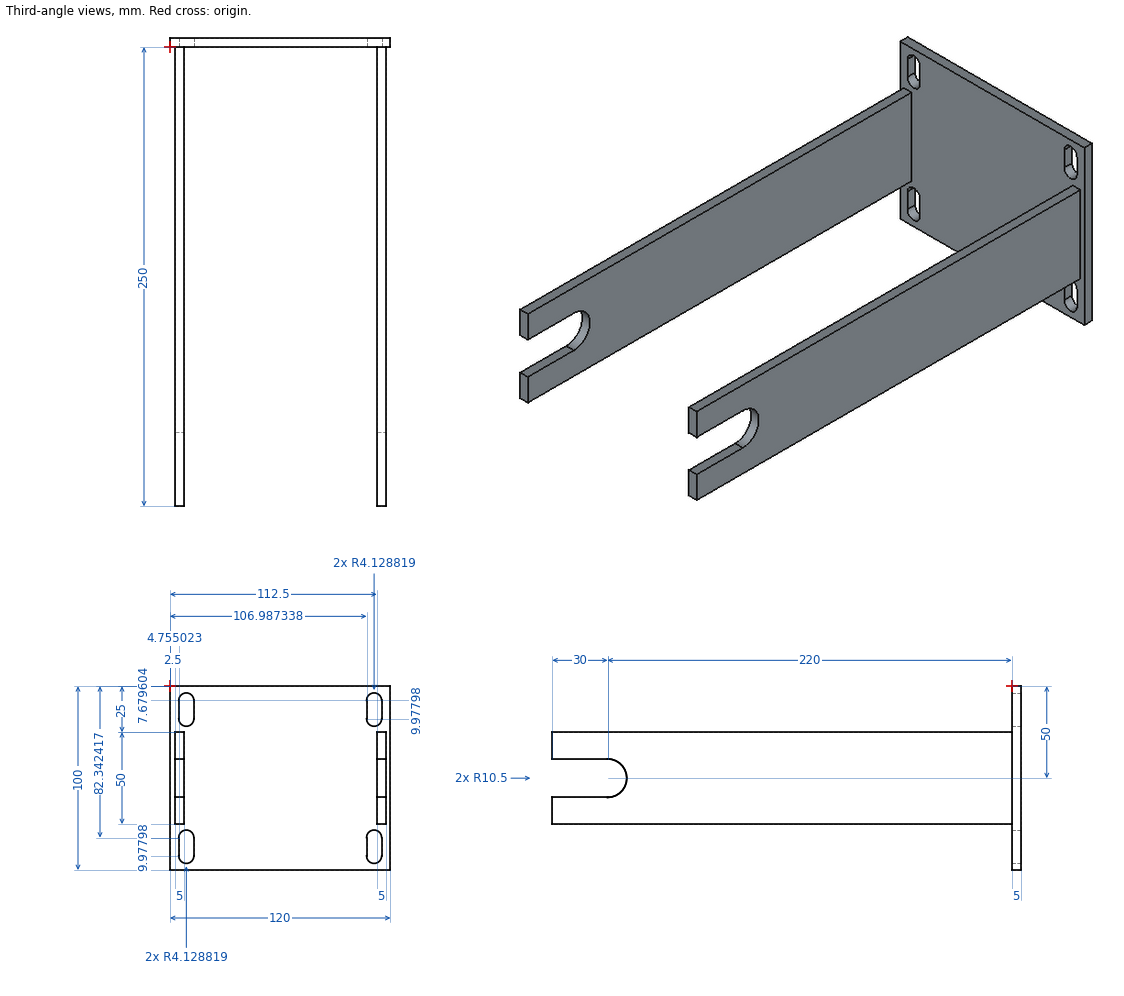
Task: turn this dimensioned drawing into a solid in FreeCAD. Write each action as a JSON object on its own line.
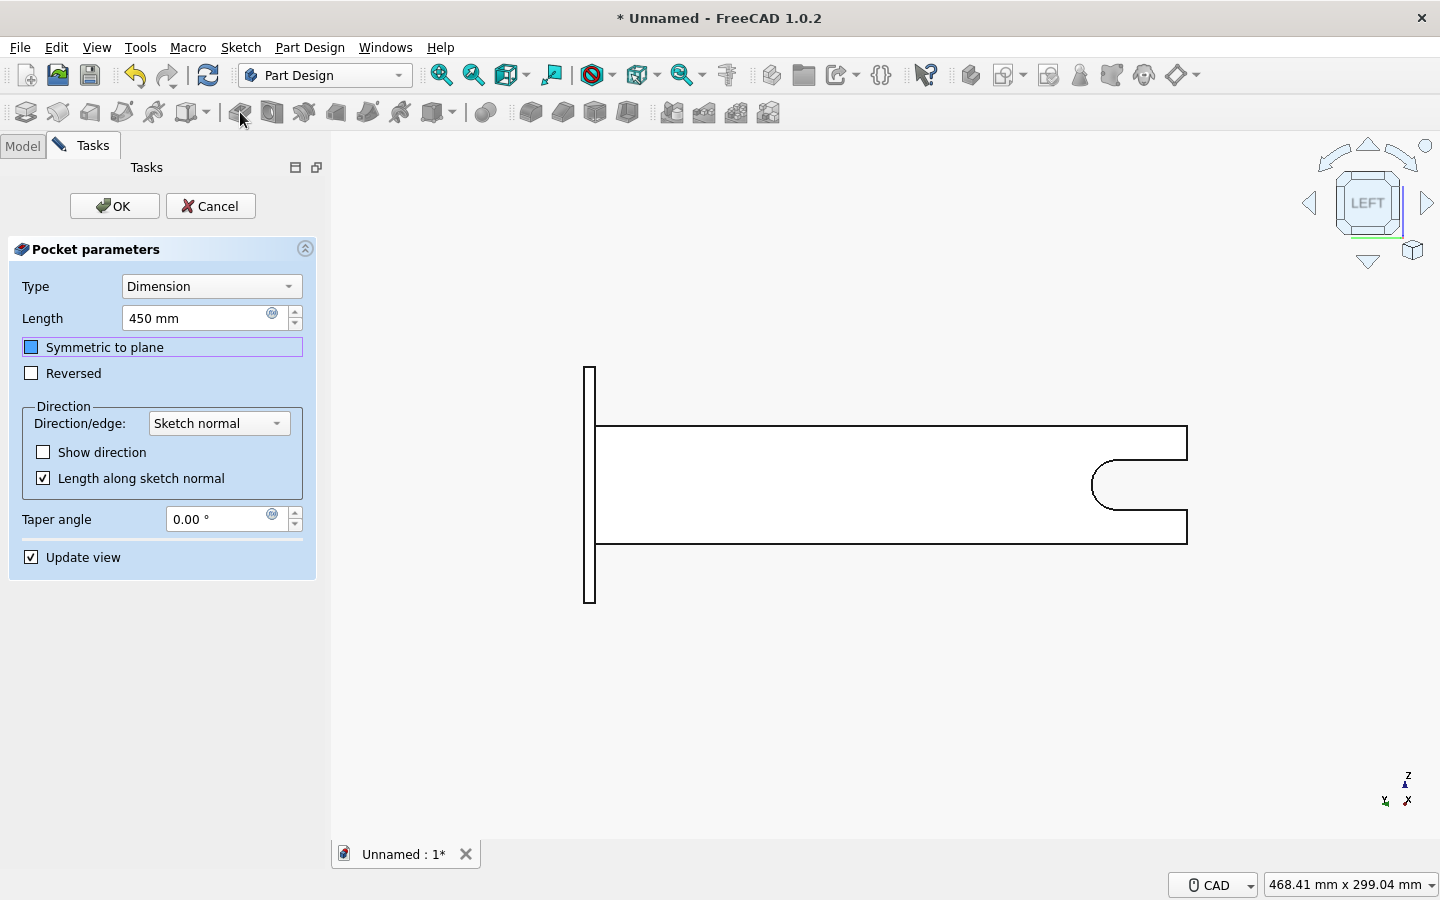
{"action": "left_click", "coordinate": [115, 206]}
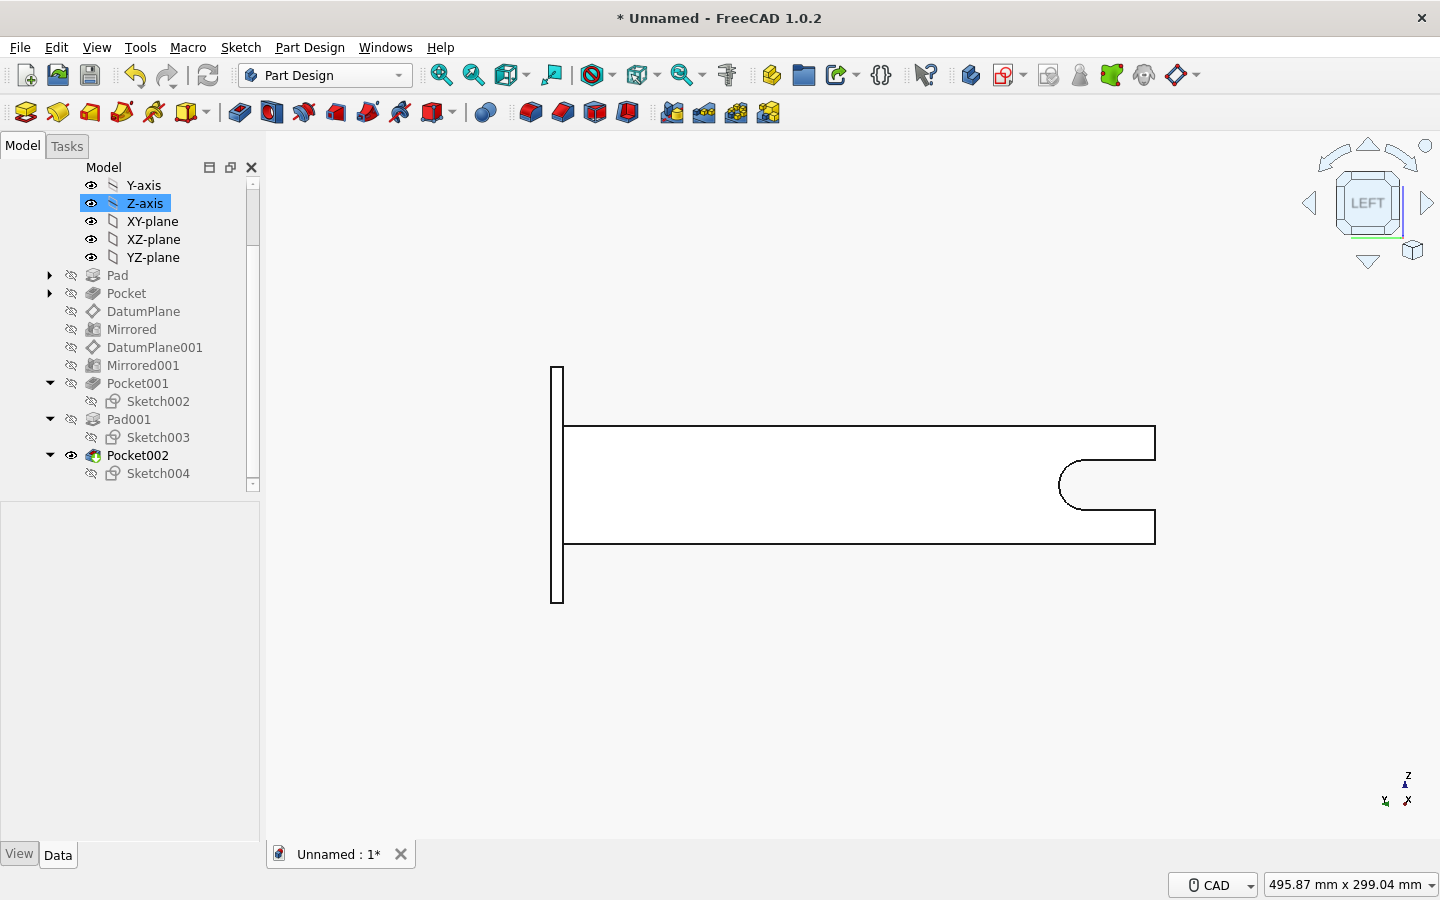
{"action": "key", "text": "0"}